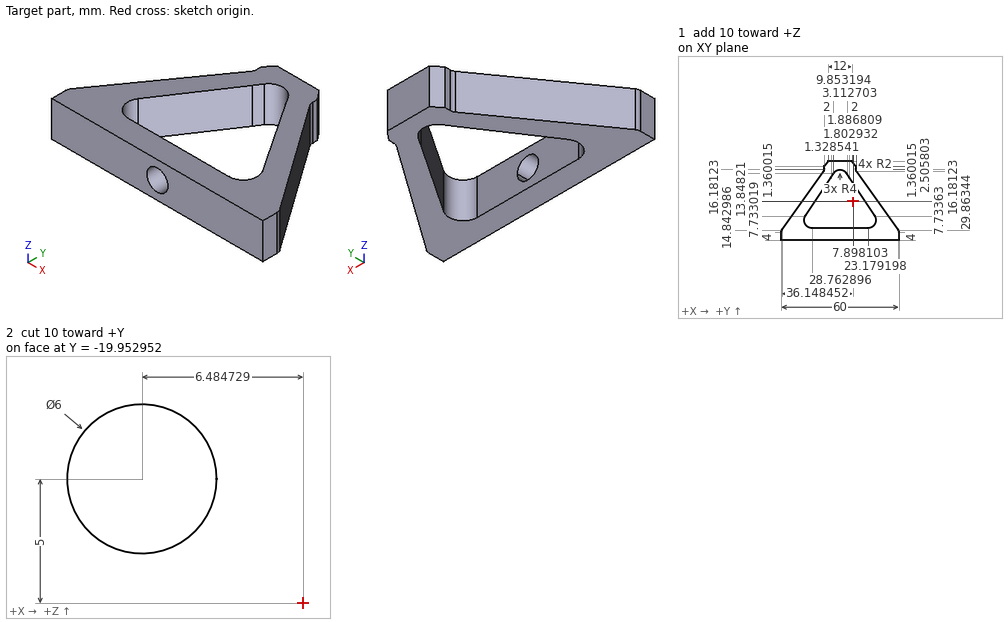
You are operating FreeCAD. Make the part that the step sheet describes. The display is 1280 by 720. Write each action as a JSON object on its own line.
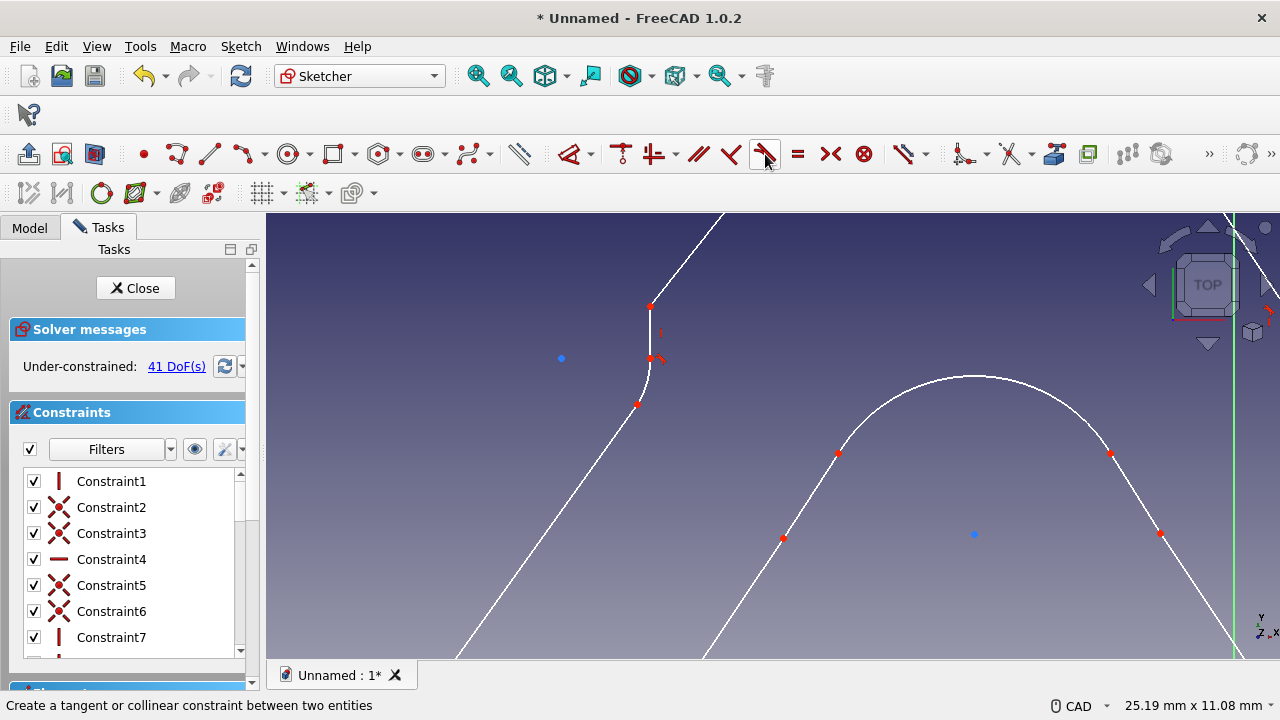
{"action": "scroll", "coordinate": [651, 324], "scroll_direction": "down", "scroll_amount": 9}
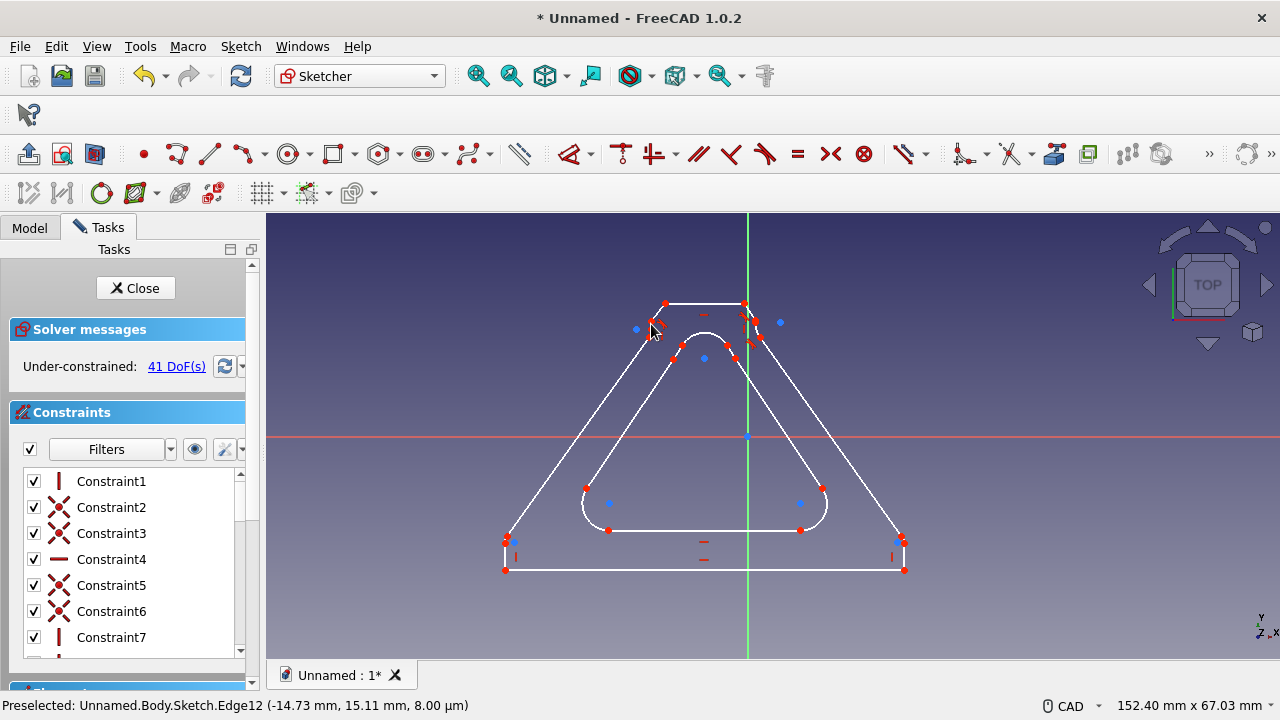
{"action": "left_click", "coordinate": [606, 397]}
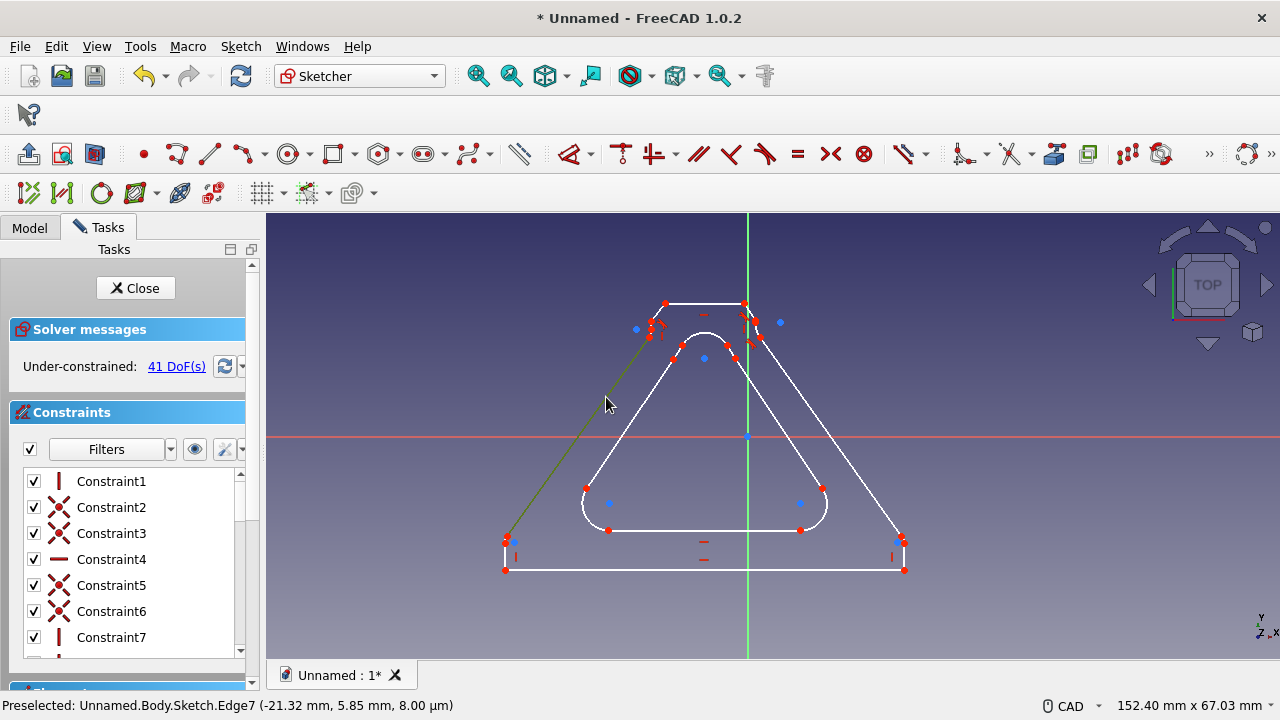
{"action": "scroll", "coordinate": [651, 334], "scroll_direction": "up", "scroll_amount": 7}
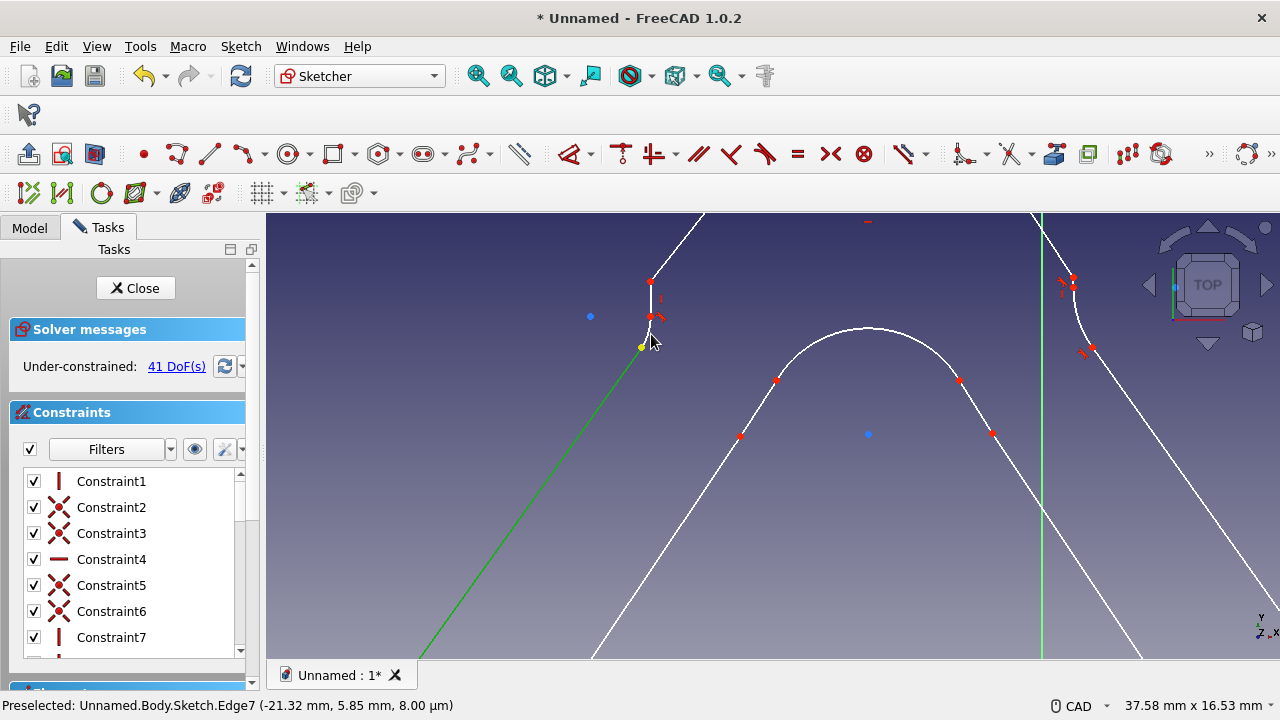
{"action": "left_click", "coordinate": [648, 333]}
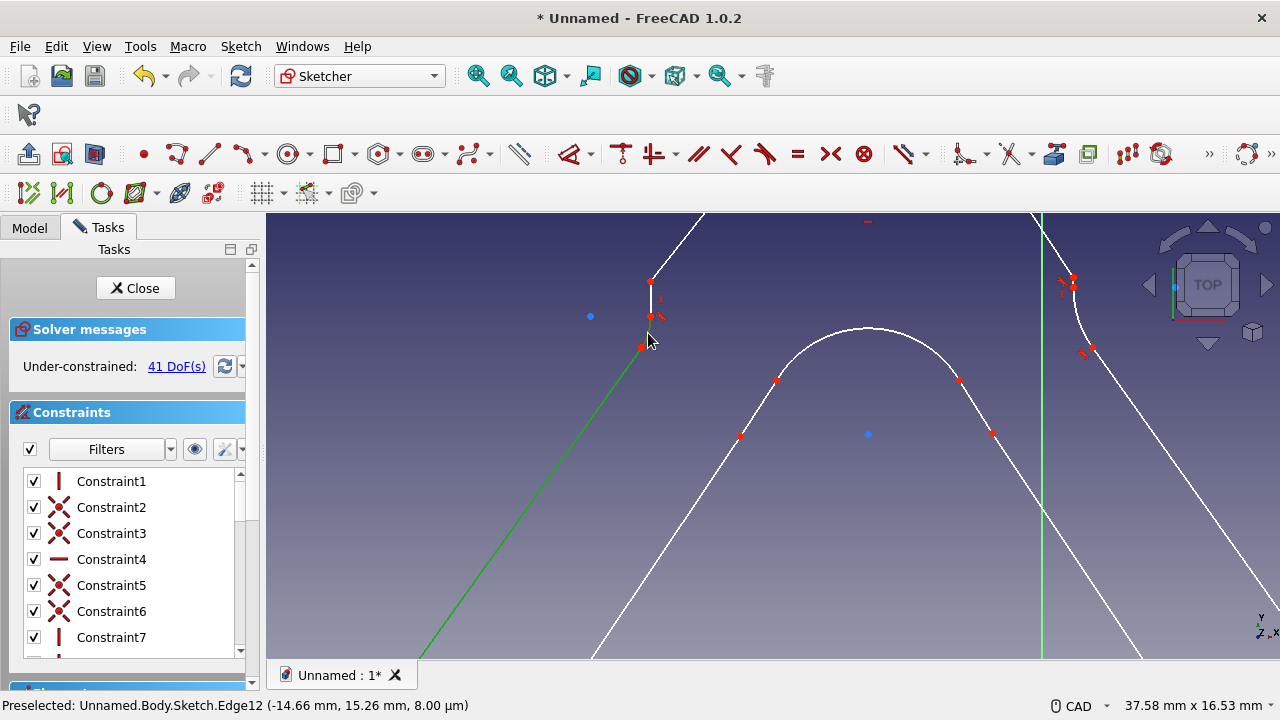
{"action": "left_click", "coordinate": [765, 154]}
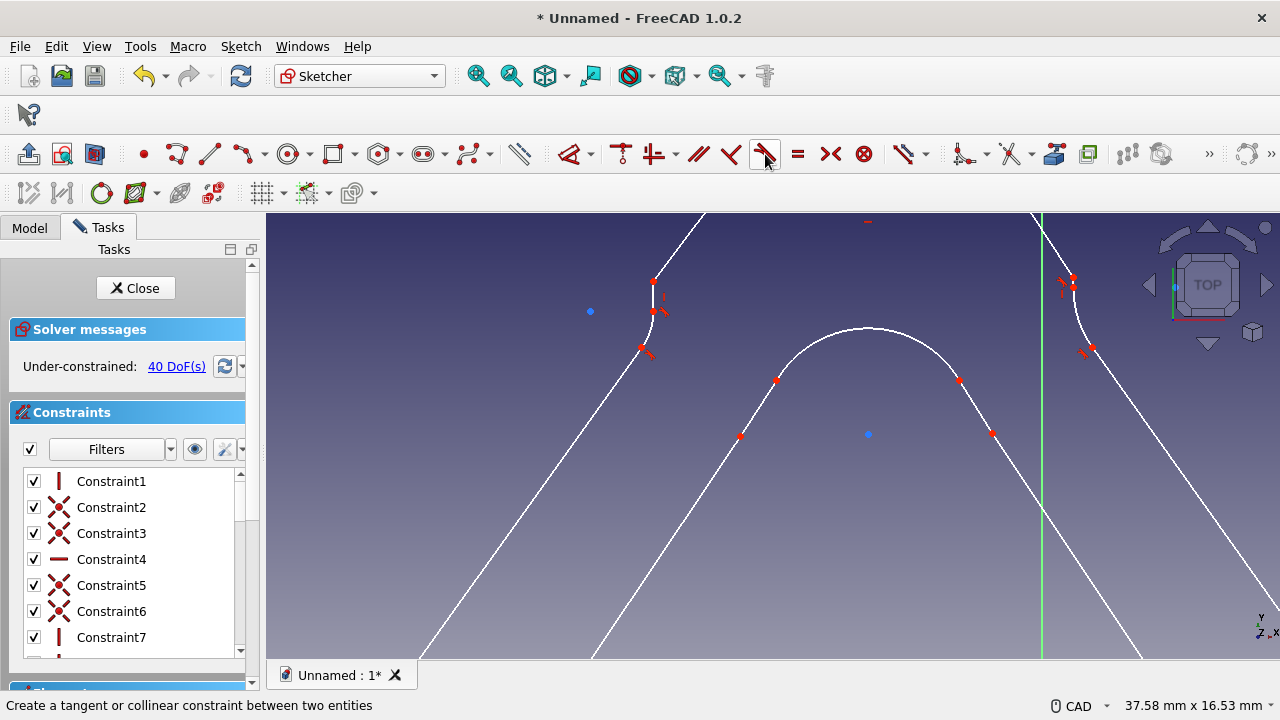
{"action": "scroll", "coordinate": [651, 334], "scroll_direction": "down", "scroll_amount": 7}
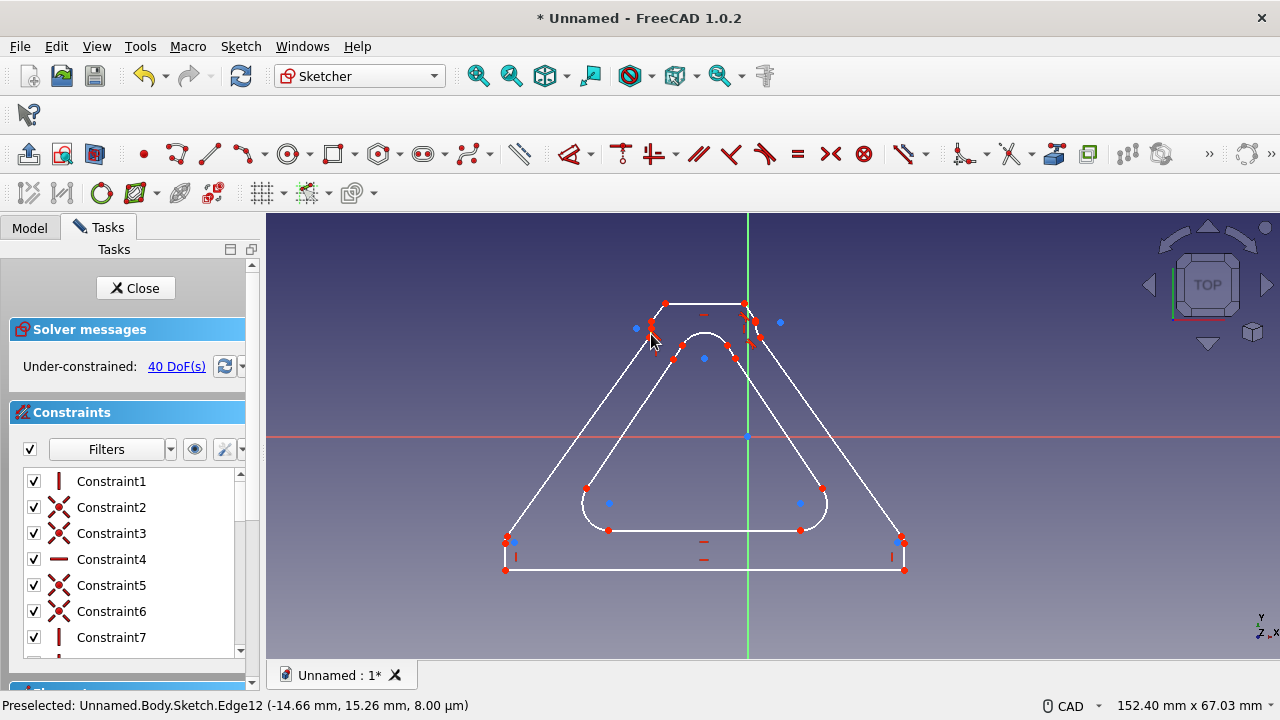
{"action": "scroll", "coordinate": [505, 552], "scroll_direction": "up", "scroll_amount": 3}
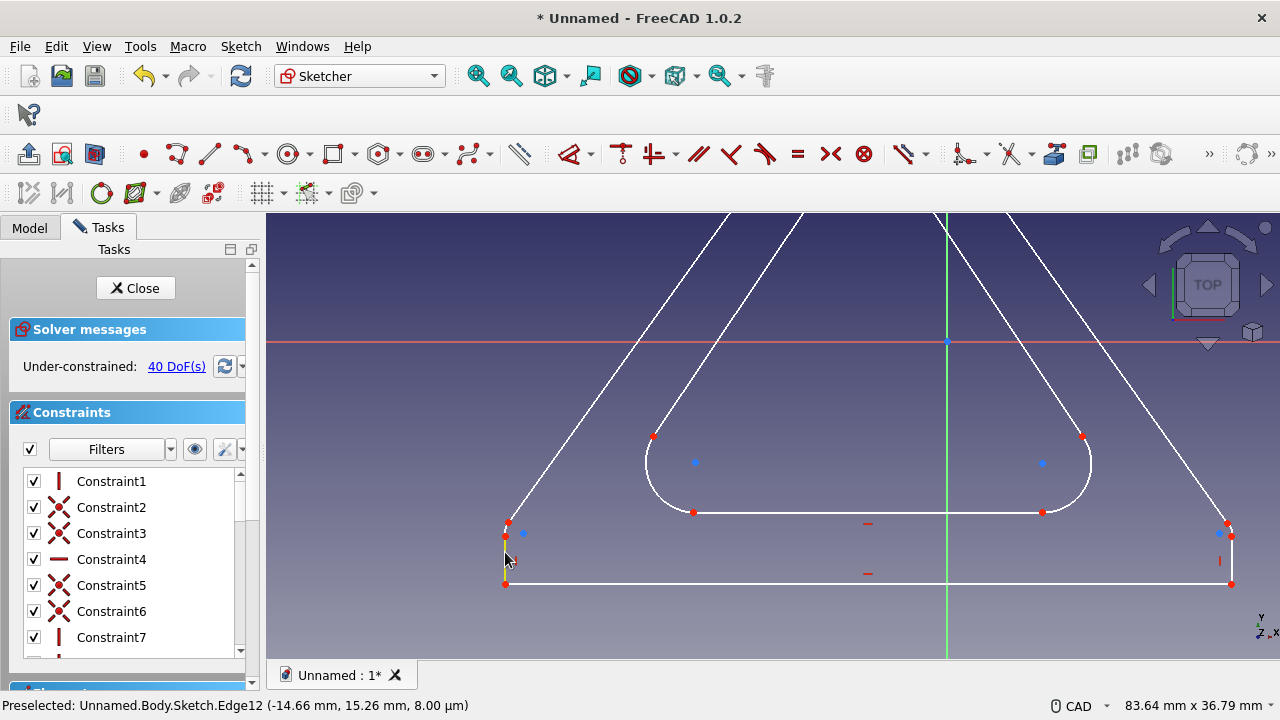
{"action": "left_click", "coordinate": [505, 551]}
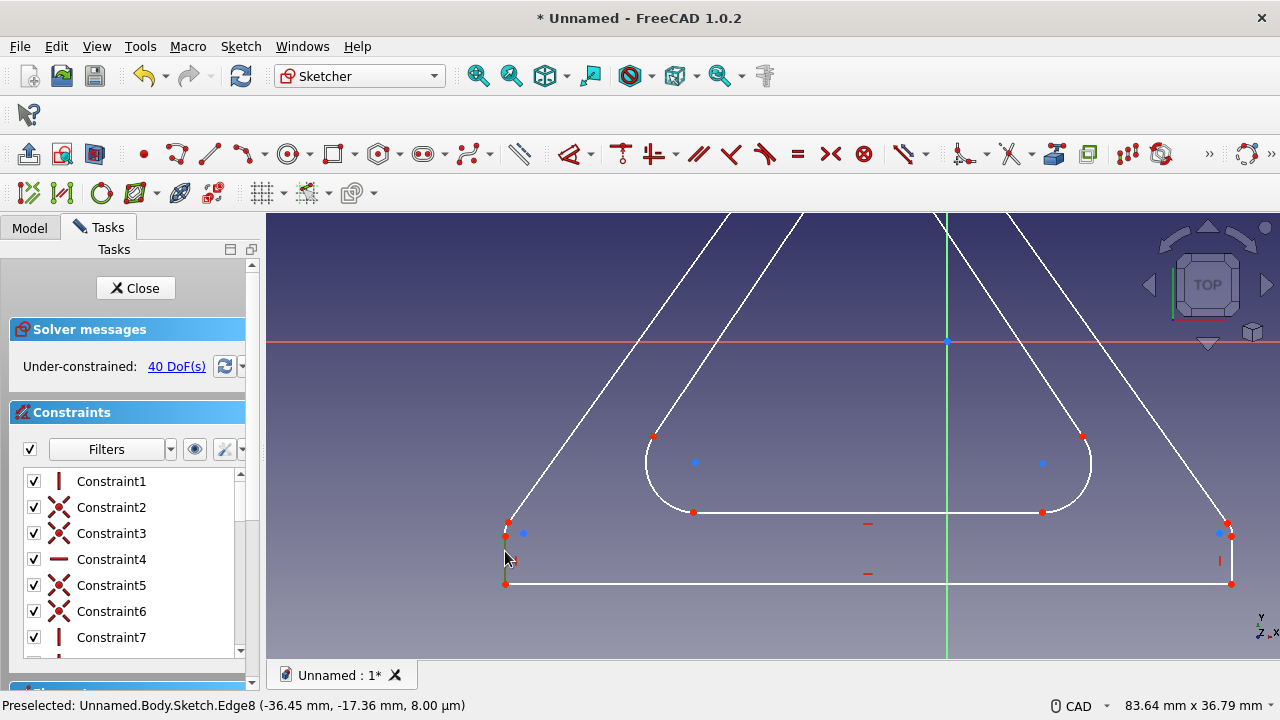
{"action": "scroll", "coordinate": [506, 529], "scroll_direction": "up", "scroll_amount": 4}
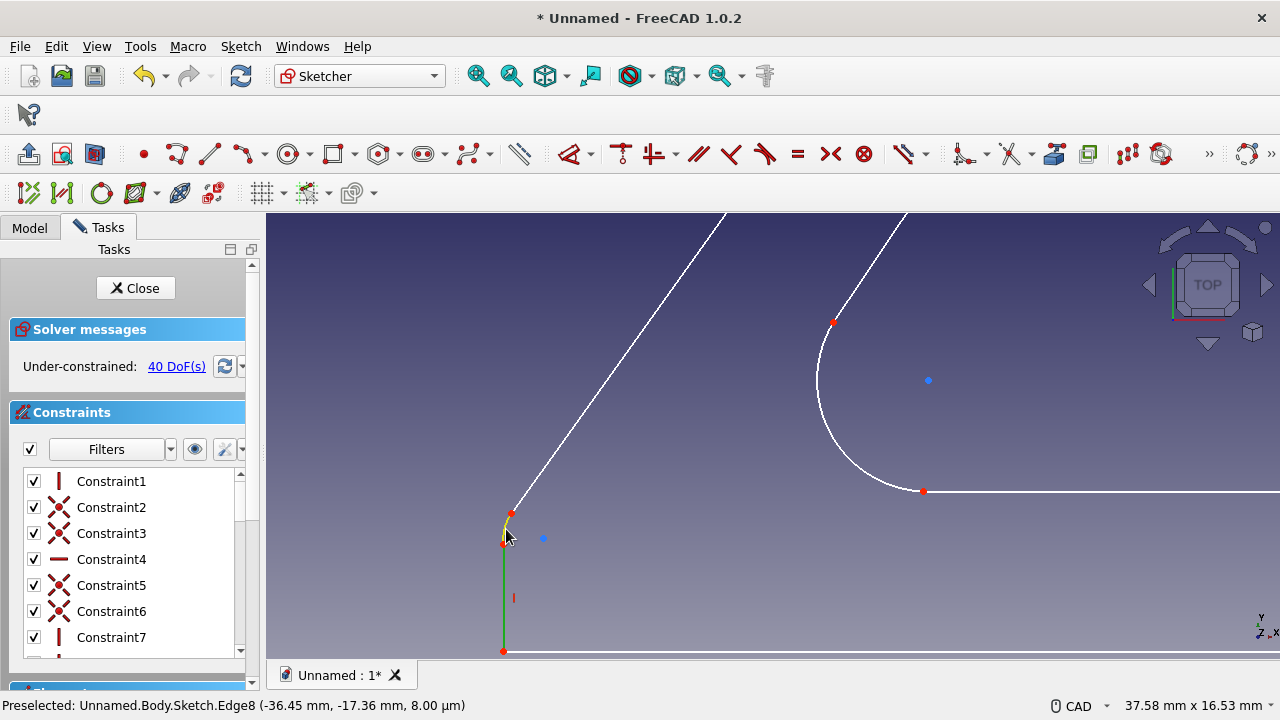
{"action": "left_click", "coordinate": [505, 528]}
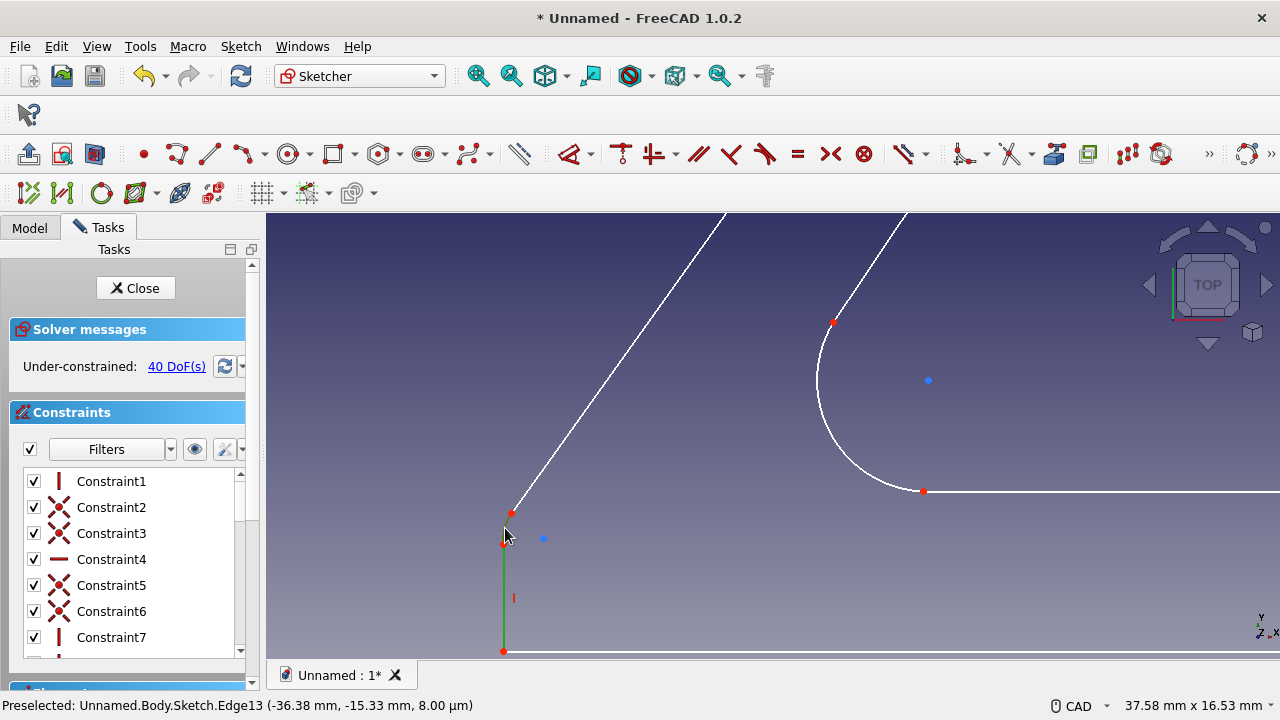
{"action": "left_click", "coordinate": [765, 154]}